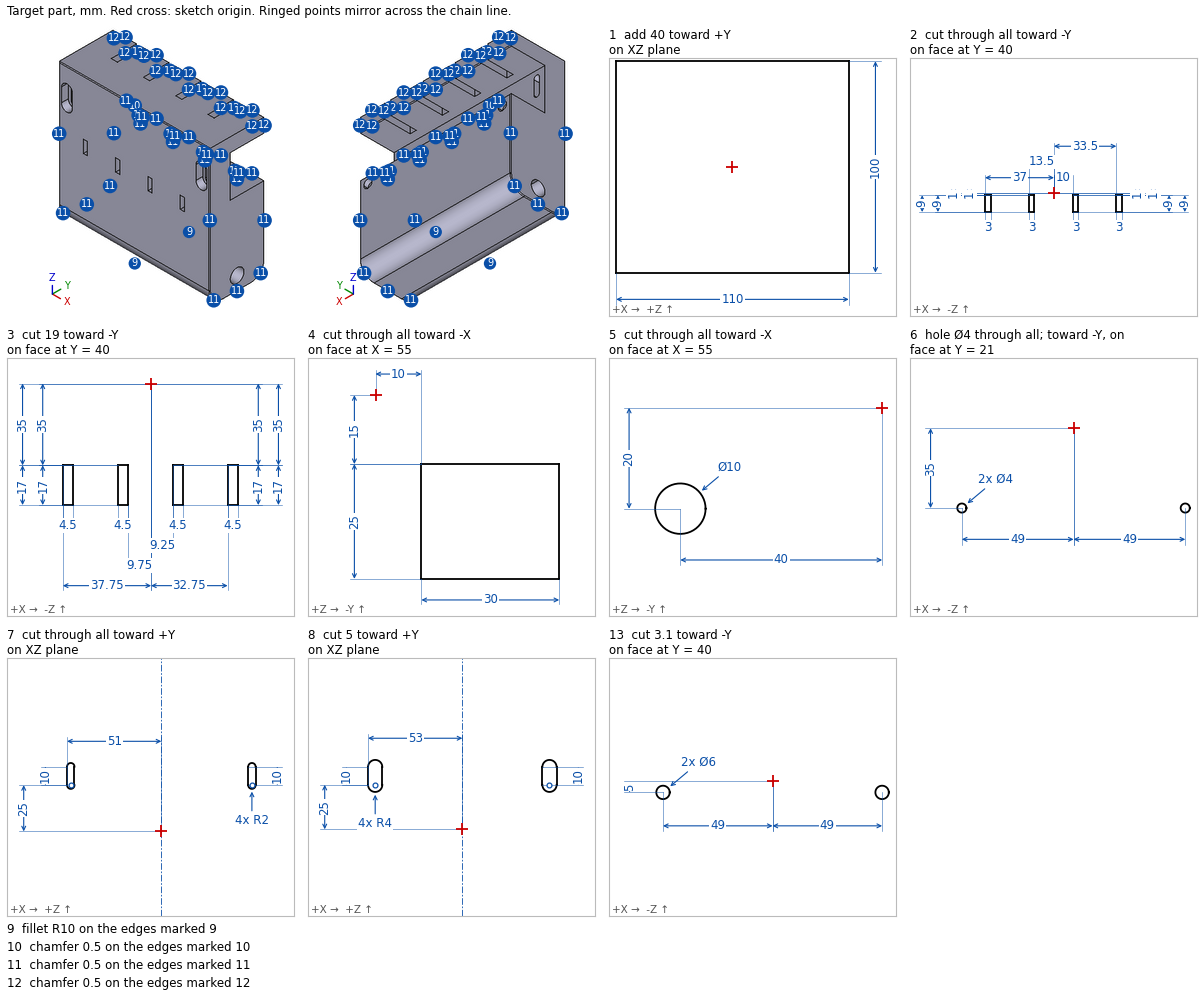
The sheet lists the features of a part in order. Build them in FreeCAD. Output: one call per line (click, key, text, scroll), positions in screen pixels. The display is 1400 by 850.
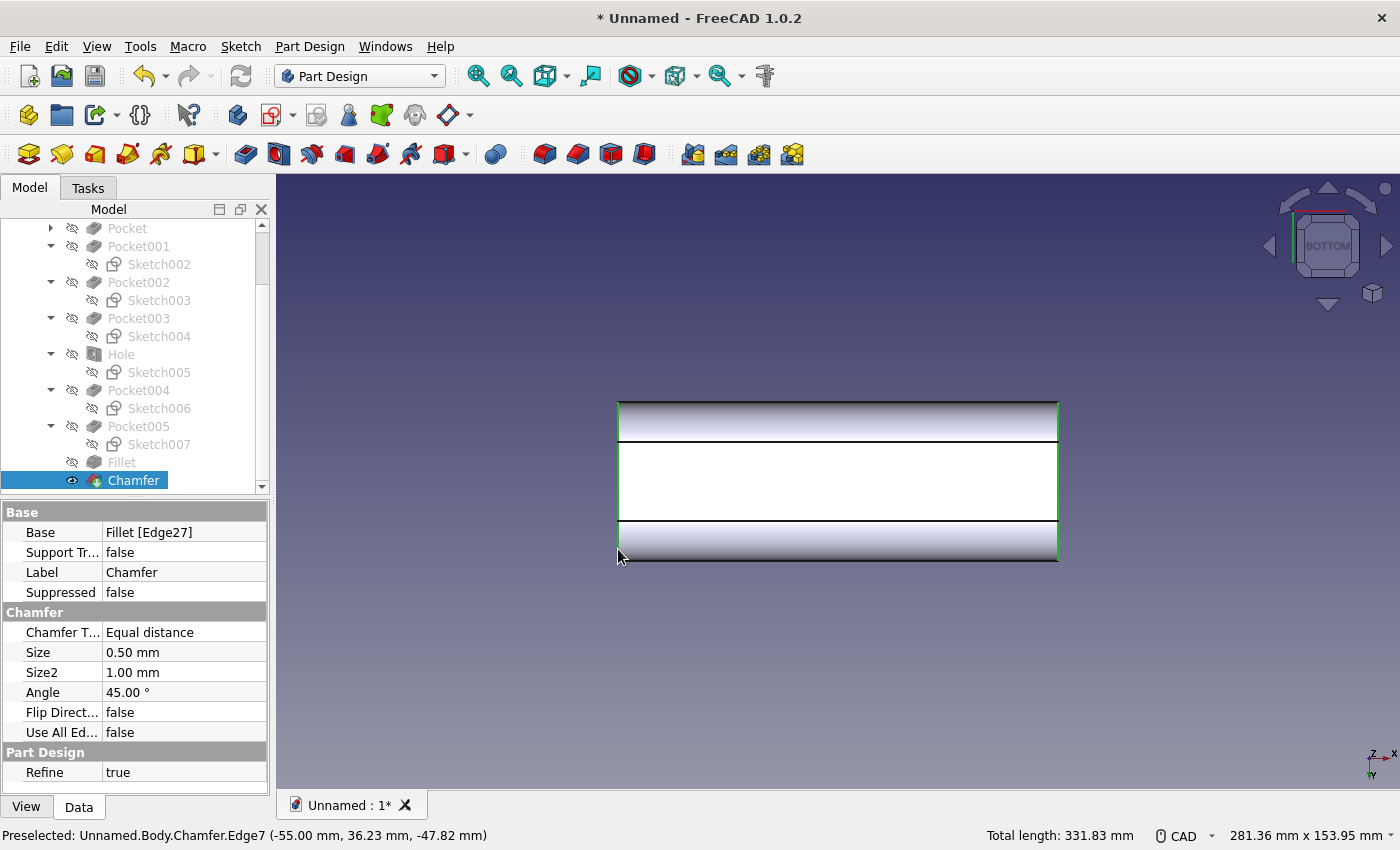
key(4)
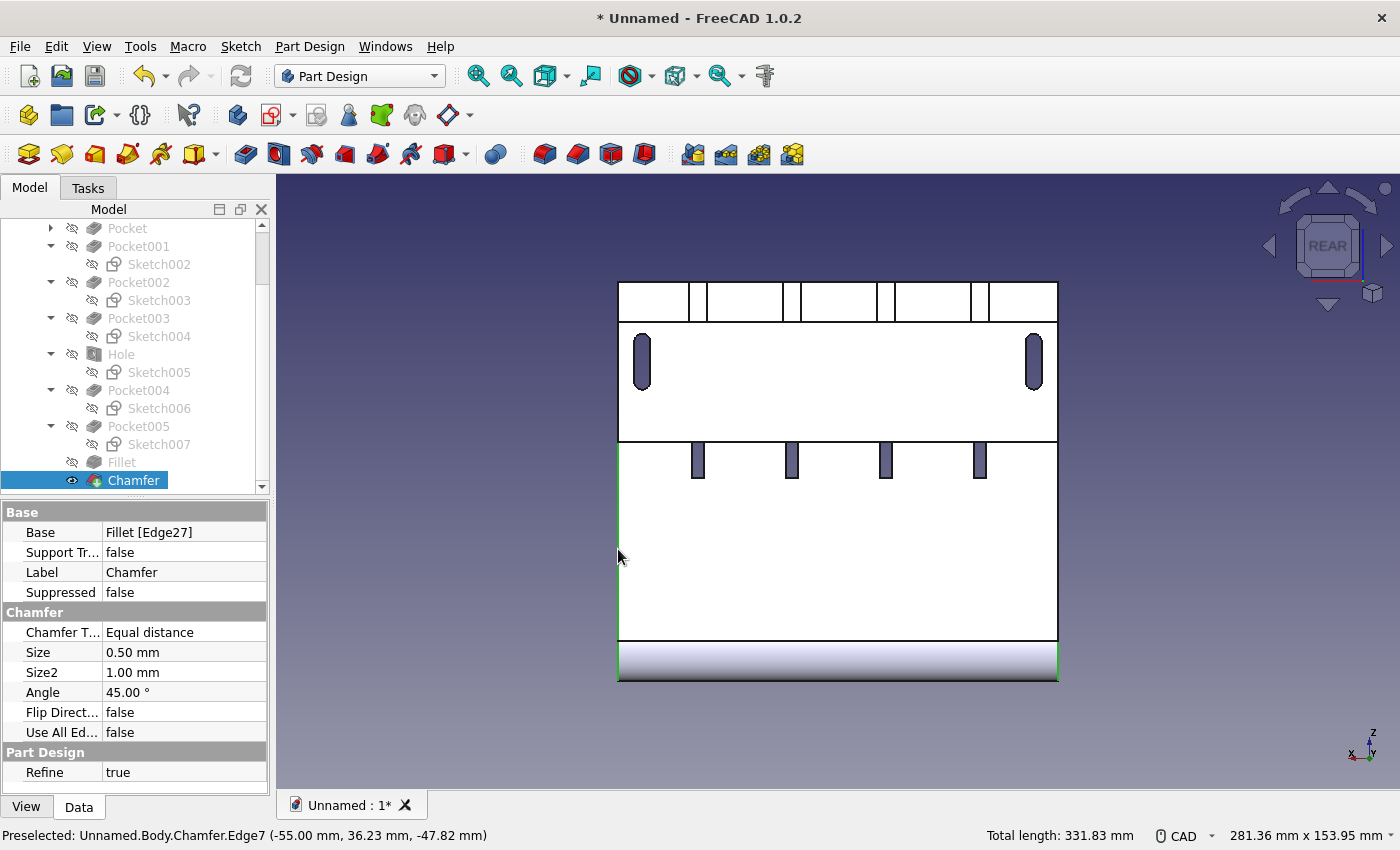
click(1058, 540, ctrl)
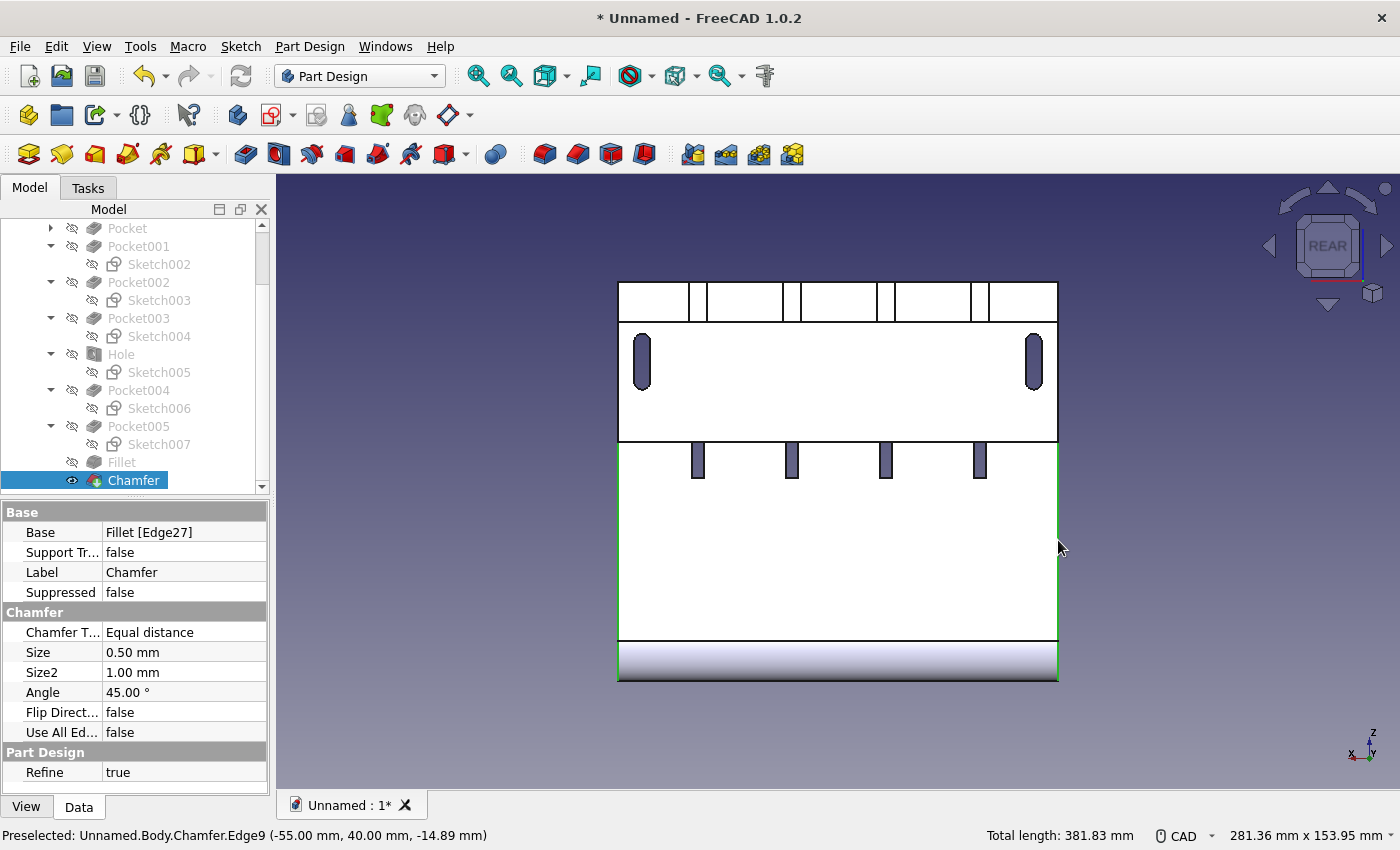
click(986, 459, ctrl)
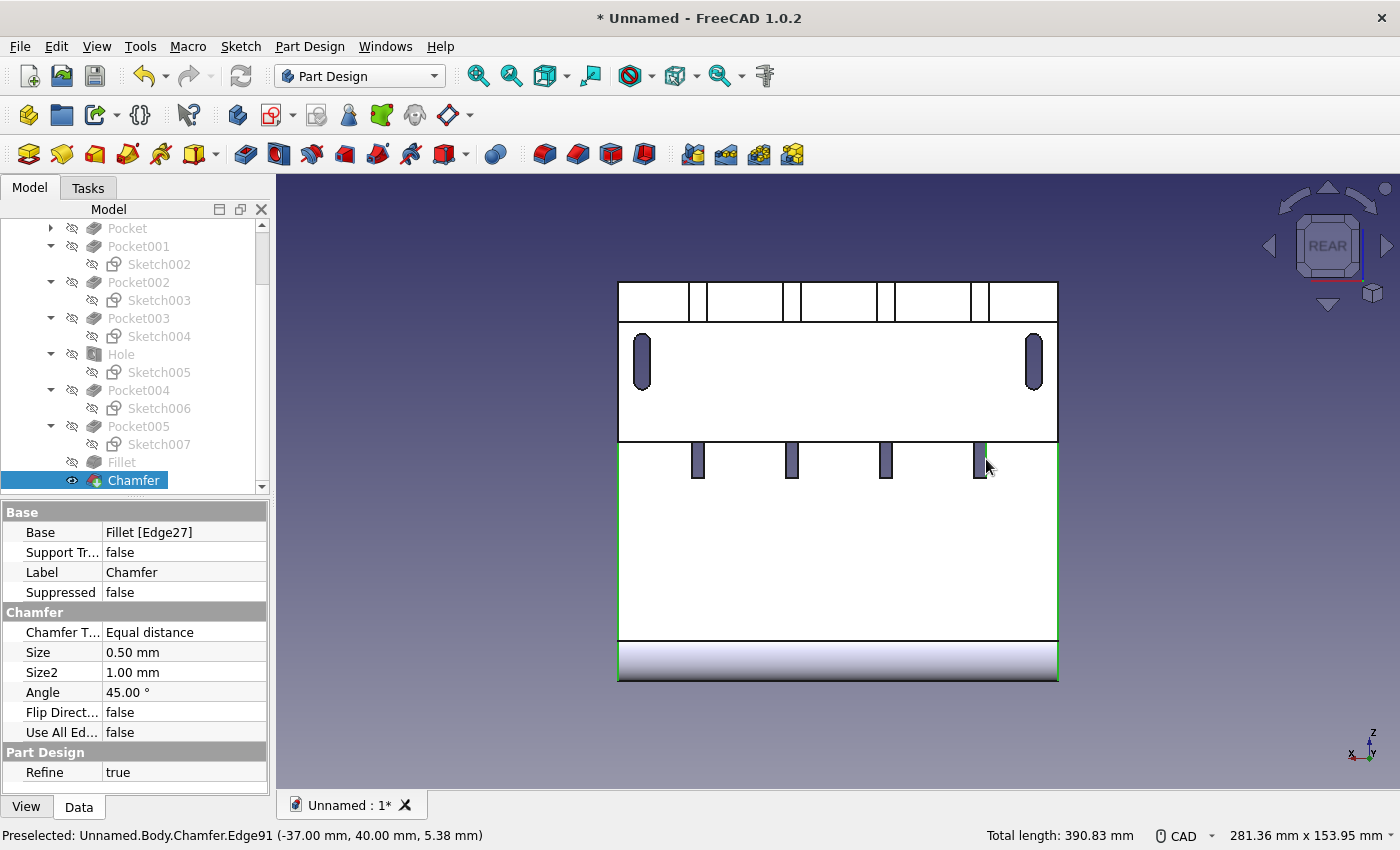
click(974, 459, ctrl)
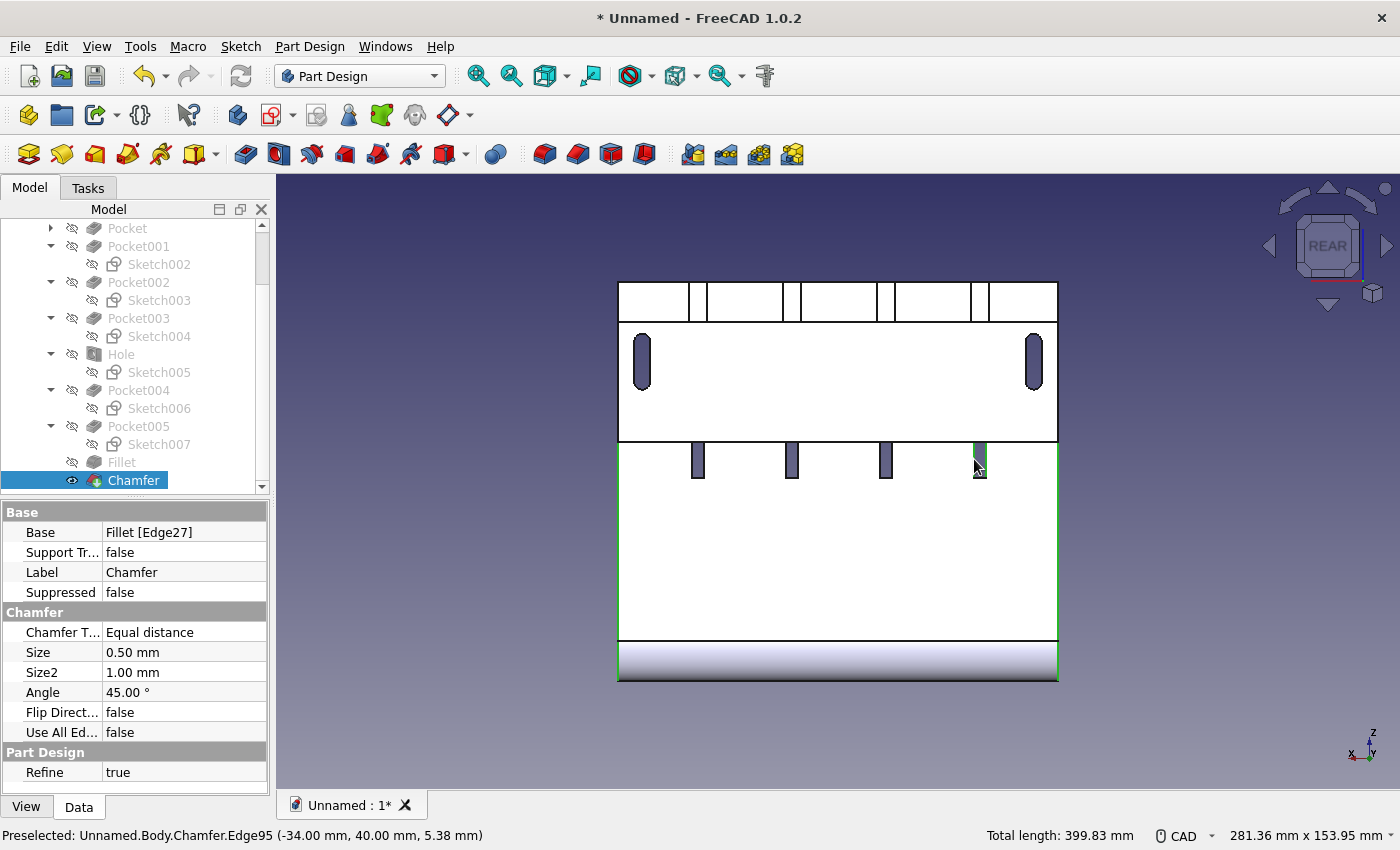
click(892, 459, ctrl)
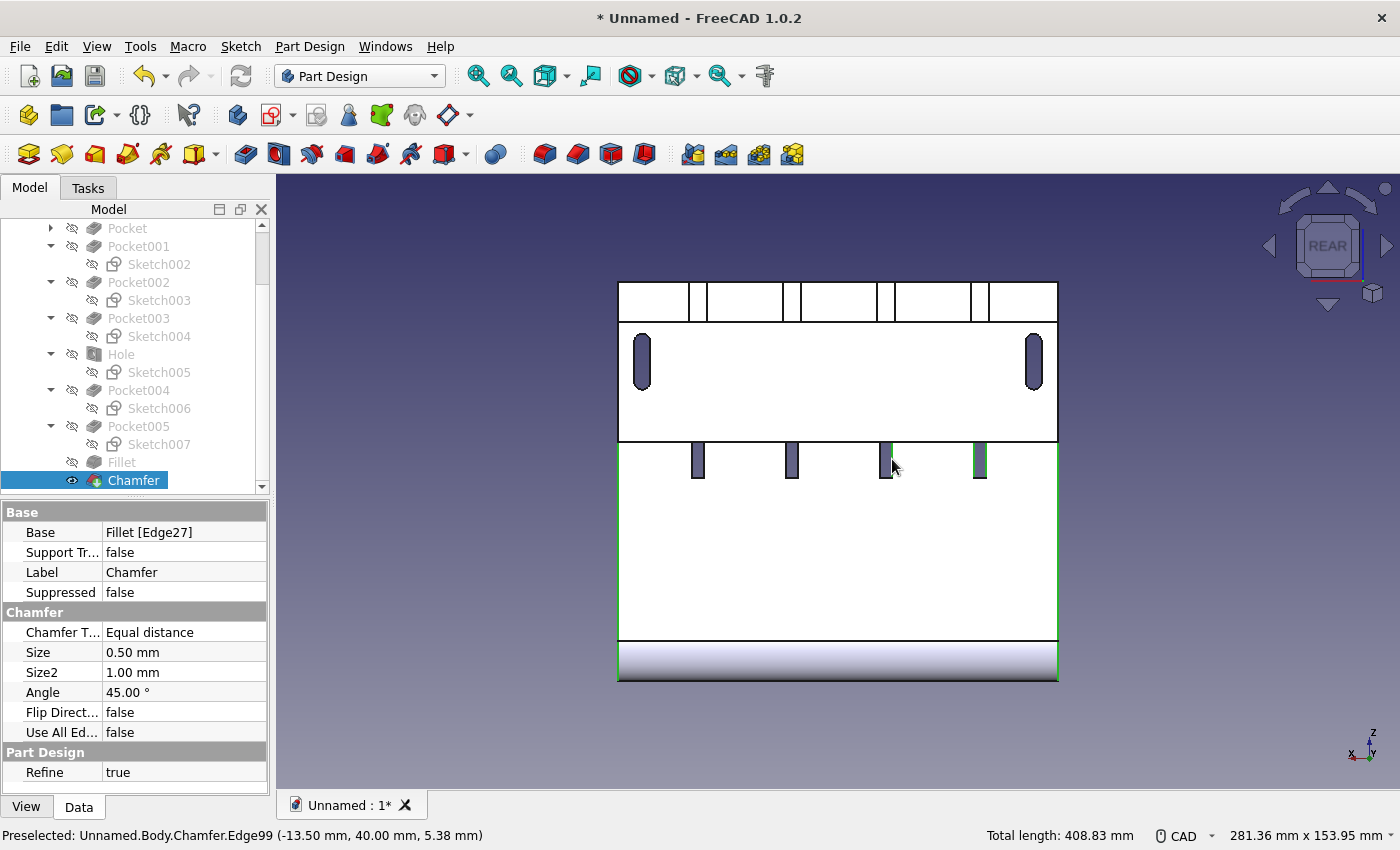
click(880, 459, ctrl)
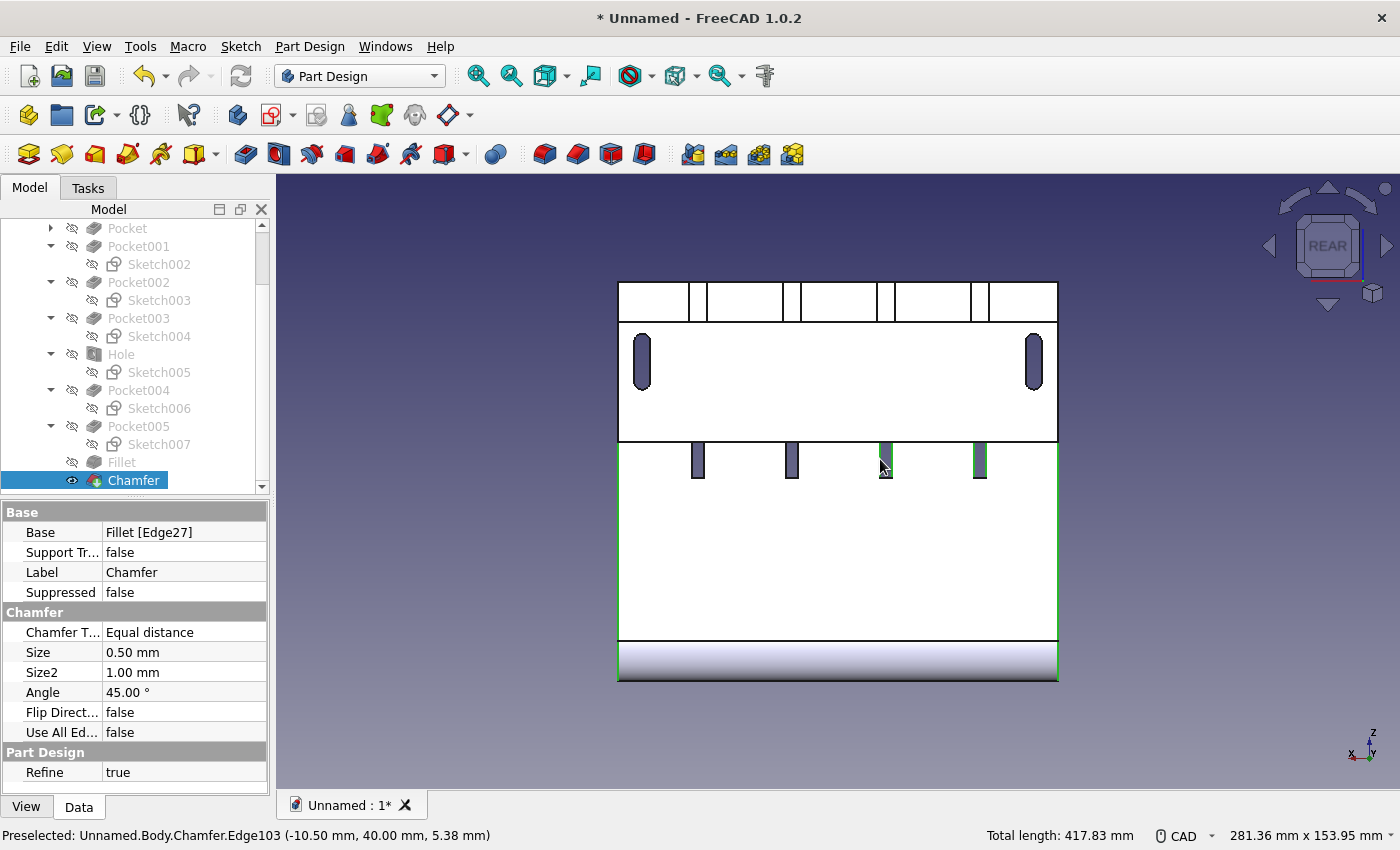
click(798, 459, ctrl)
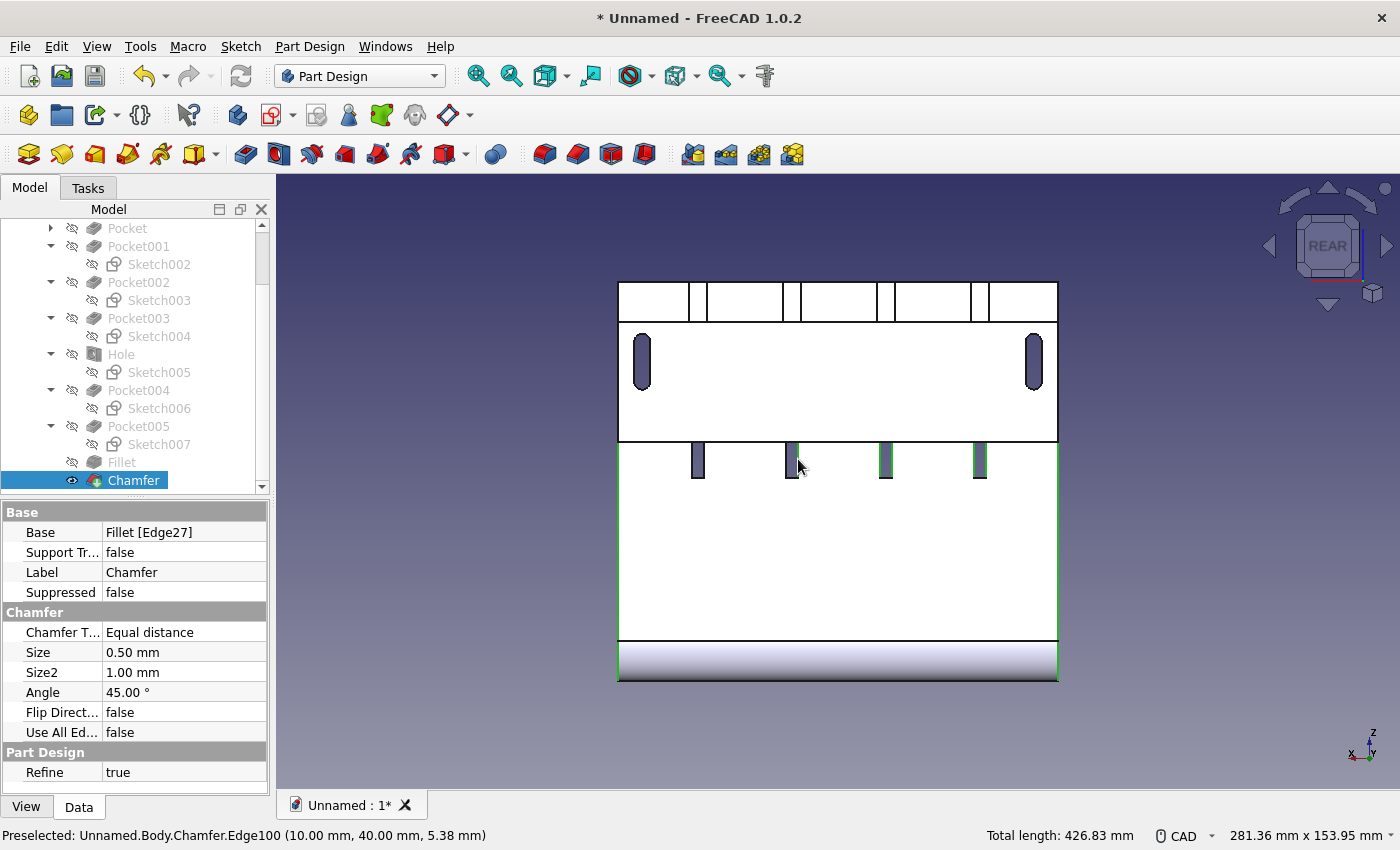
click(786, 459, ctrl)